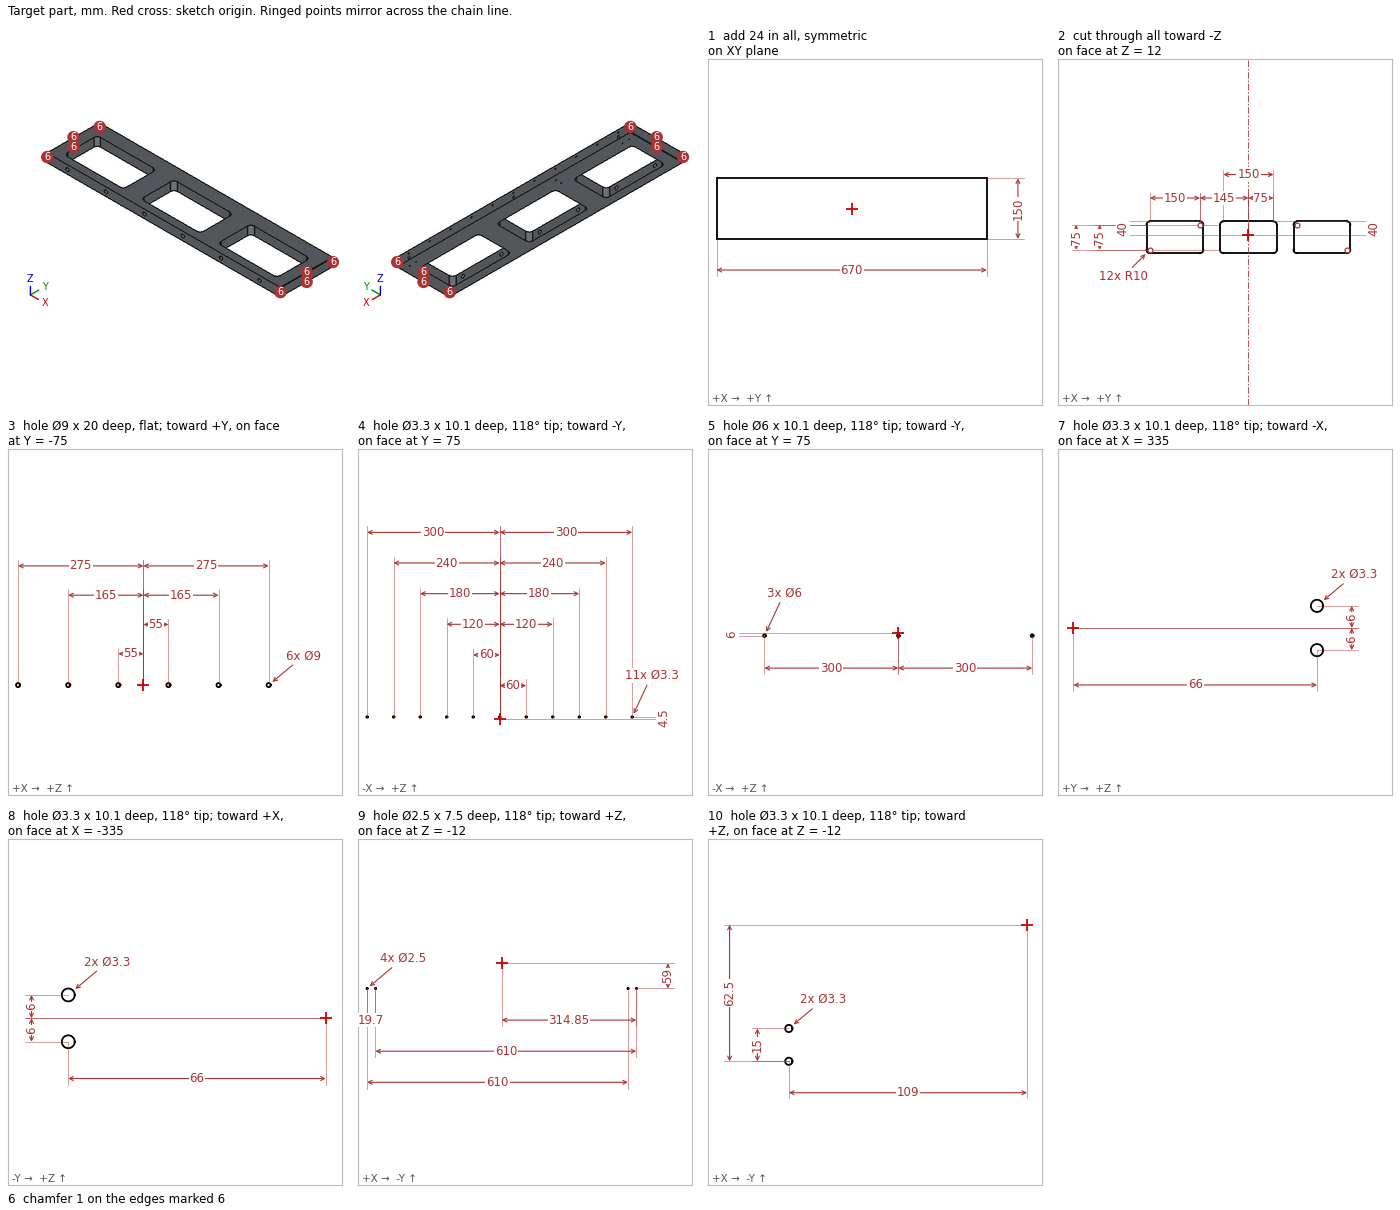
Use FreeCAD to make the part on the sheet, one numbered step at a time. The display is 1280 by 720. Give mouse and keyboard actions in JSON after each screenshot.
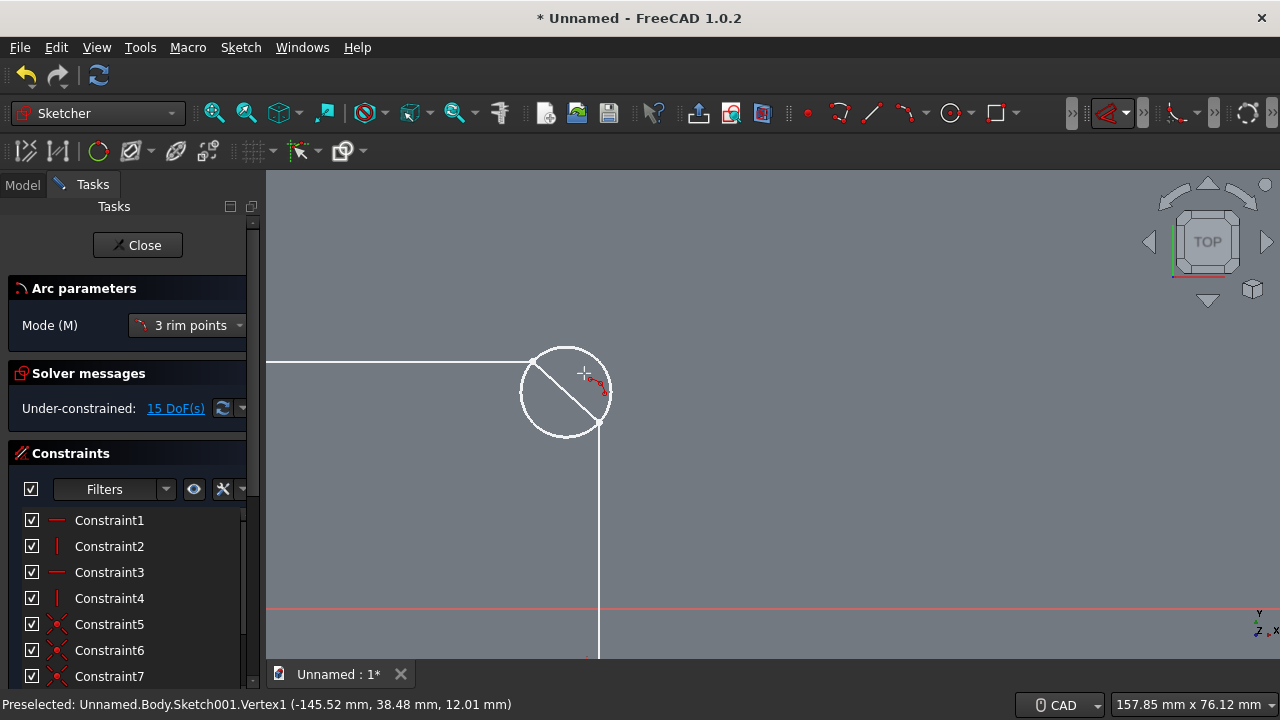
{"action": "left_click", "coordinate": [581, 371]}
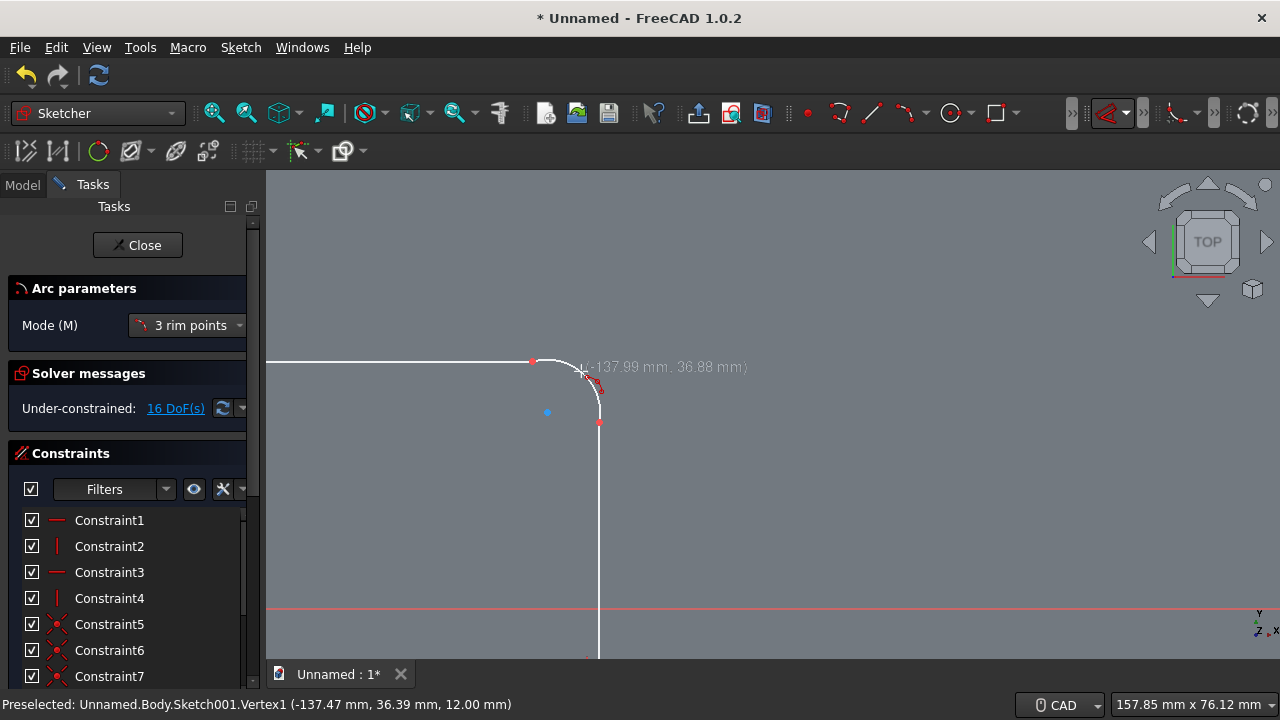
{"action": "left_click", "coordinate": [872, 114]}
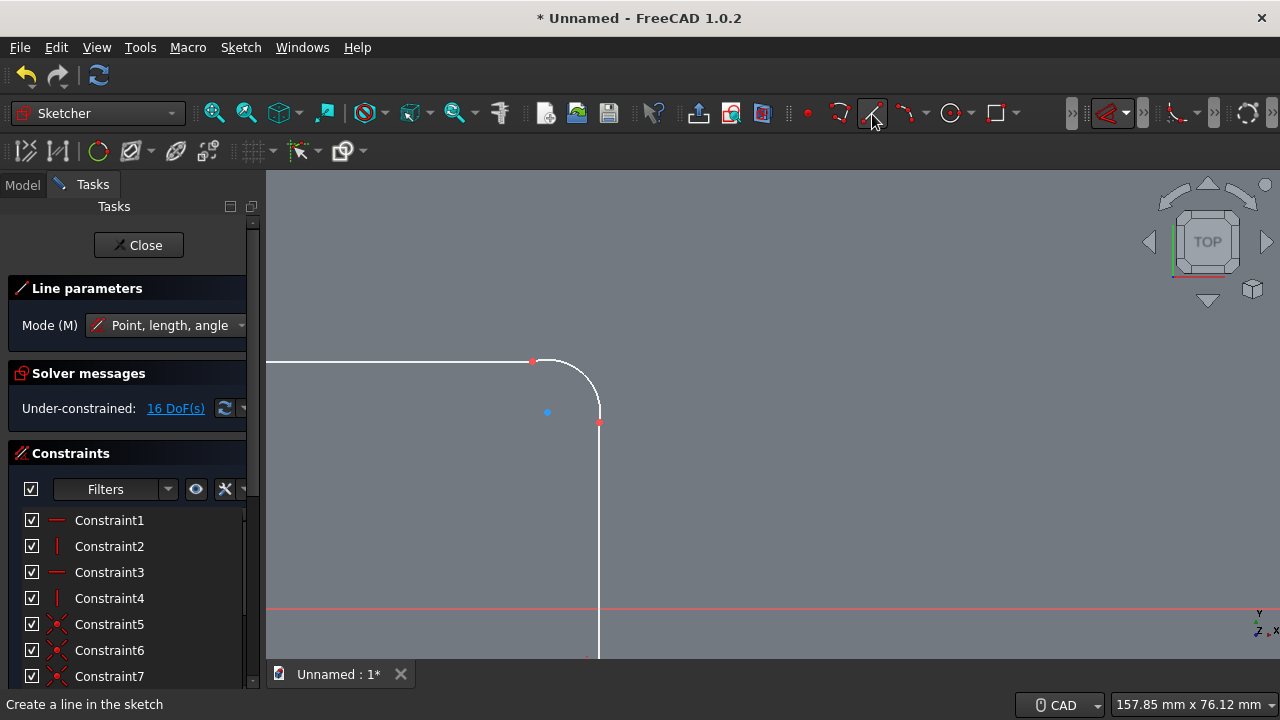
{"action": "scroll", "coordinate": [585, 377], "scroll_direction": "down", "scroll_amount": 10}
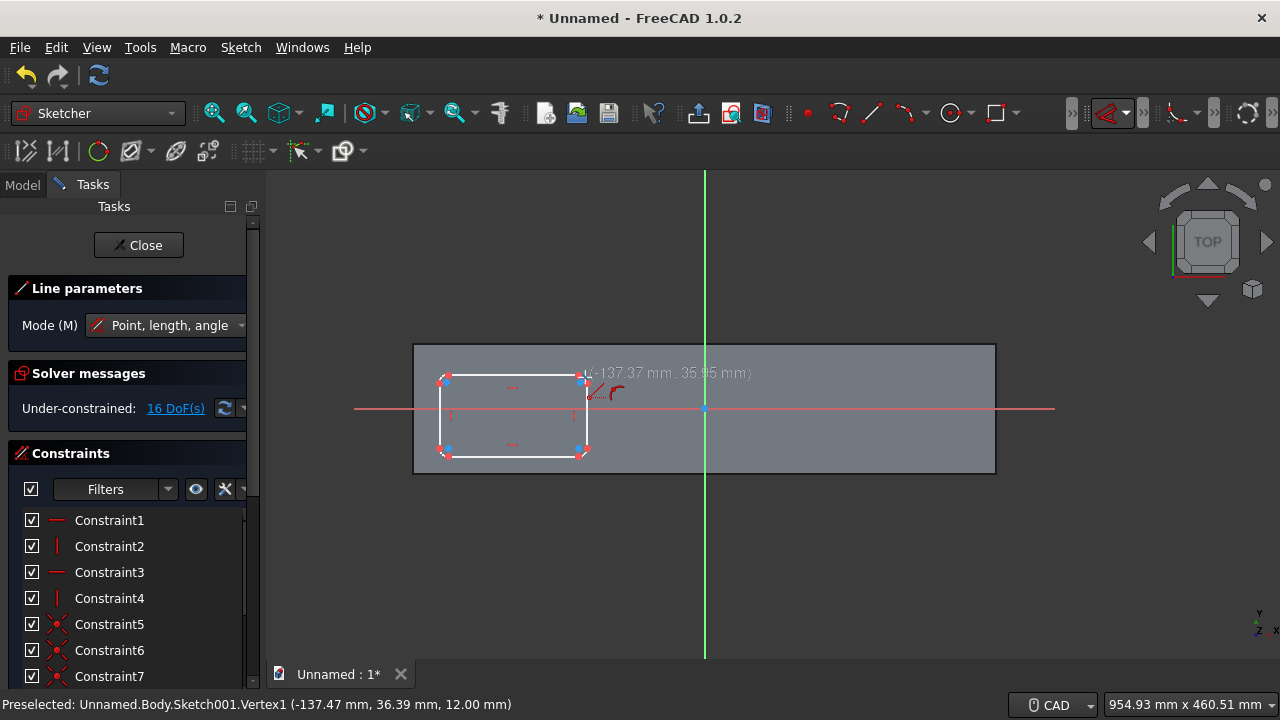
{"action": "left_click", "coordinate": [770, 374]}
{"action": "left_click", "coordinate": [639, 374]}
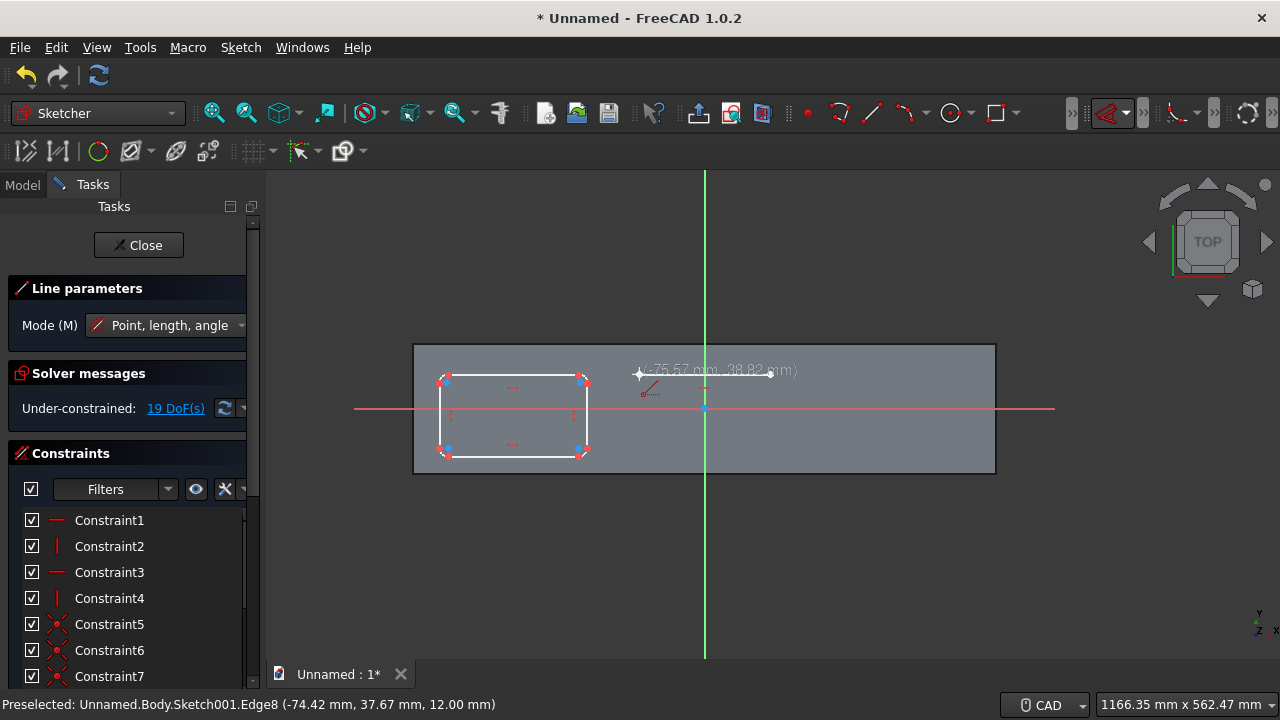
{"action": "scroll", "coordinate": [631, 383], "scroll_direction": "up", "scroll_amount": 2}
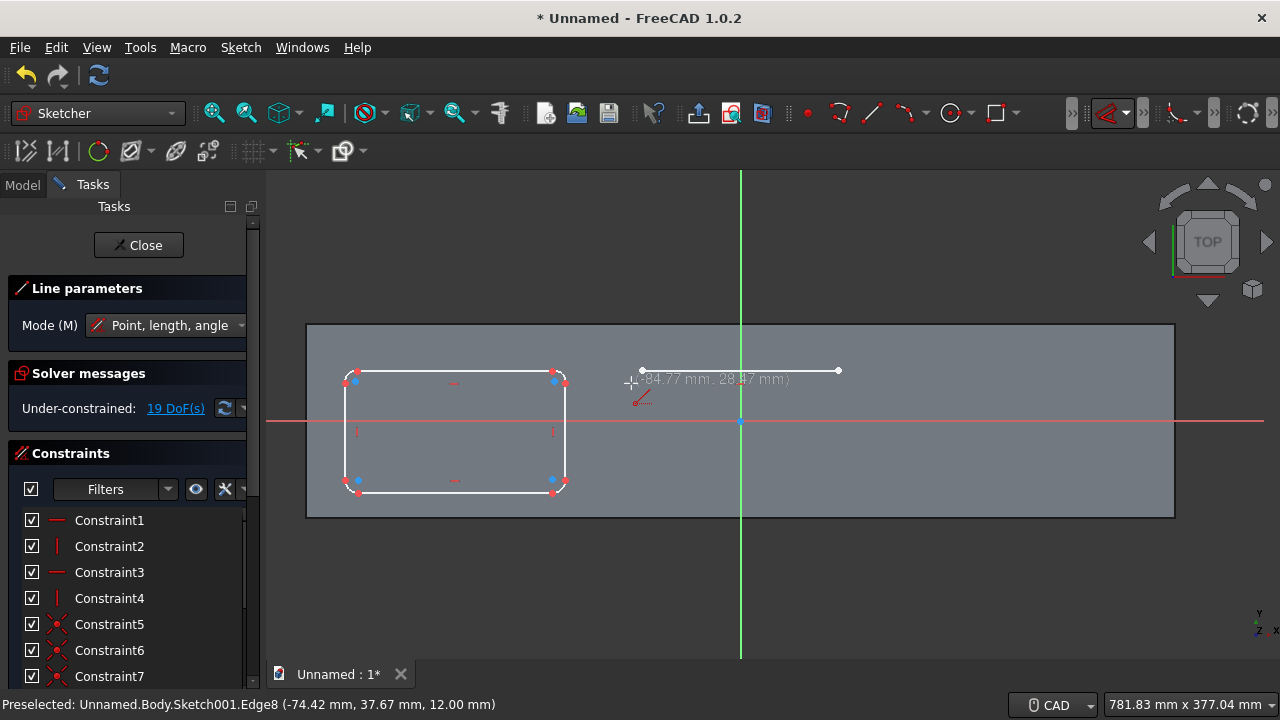
{"action": "left_click", "coordinate": [631, 382]}
{"action": "left_click", "coordinate": [631, 480]}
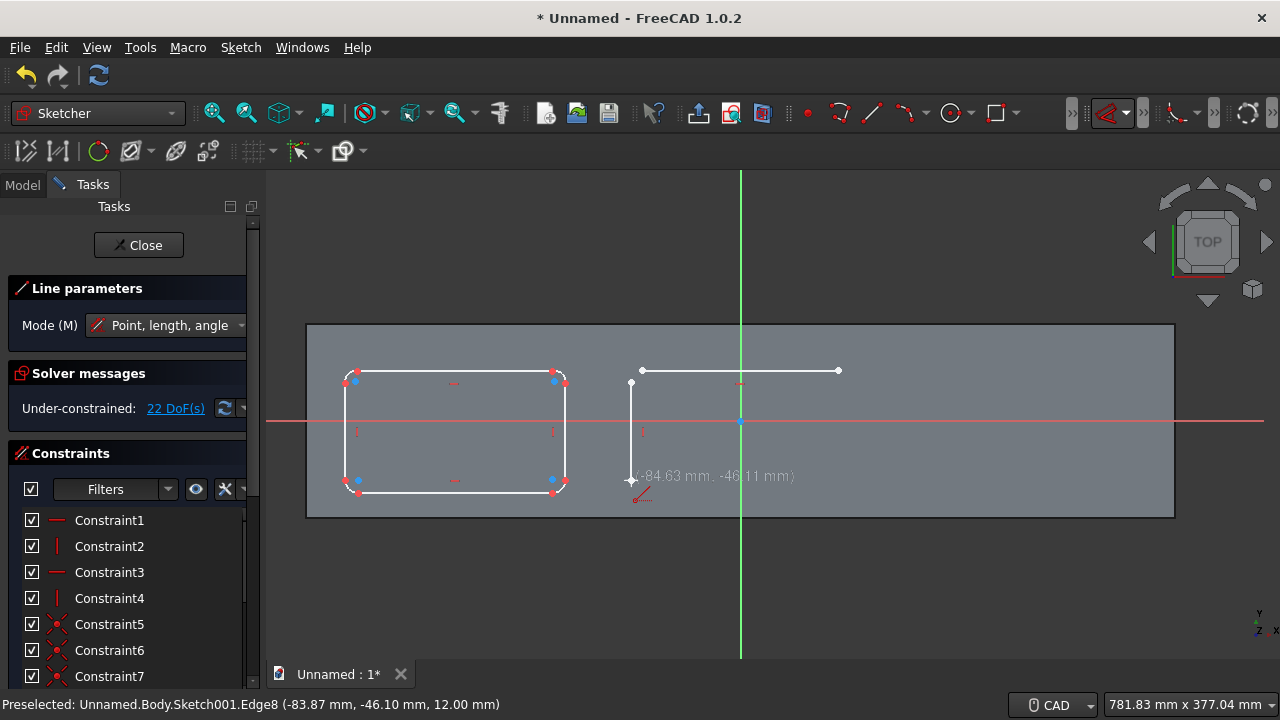
{"action": "left_click", "coordinate": [643, 493]}
{"action": "left_click", "coordinate": [838, 493]}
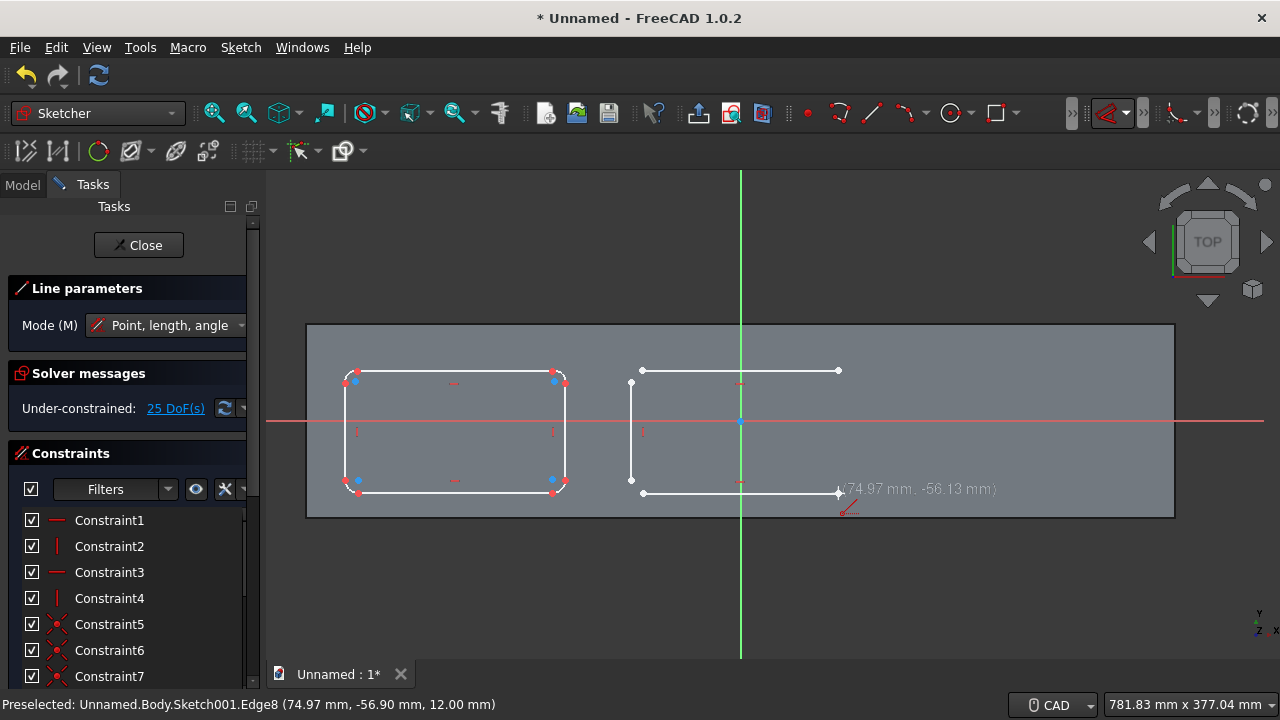
{"action": "left_click", "coordinate": [851, 480]}
{"action": "left_click", "coordinate": [851, 382]}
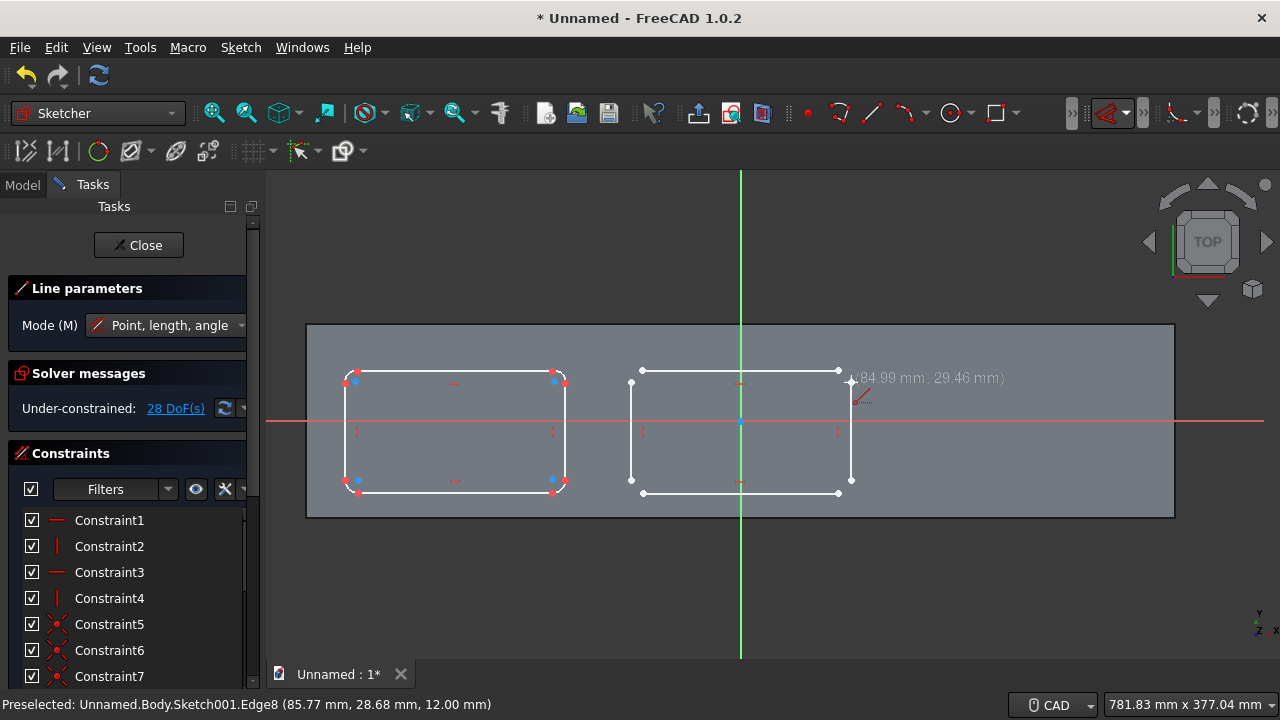
{"action": "left_click", "coordinate": [906, 114]}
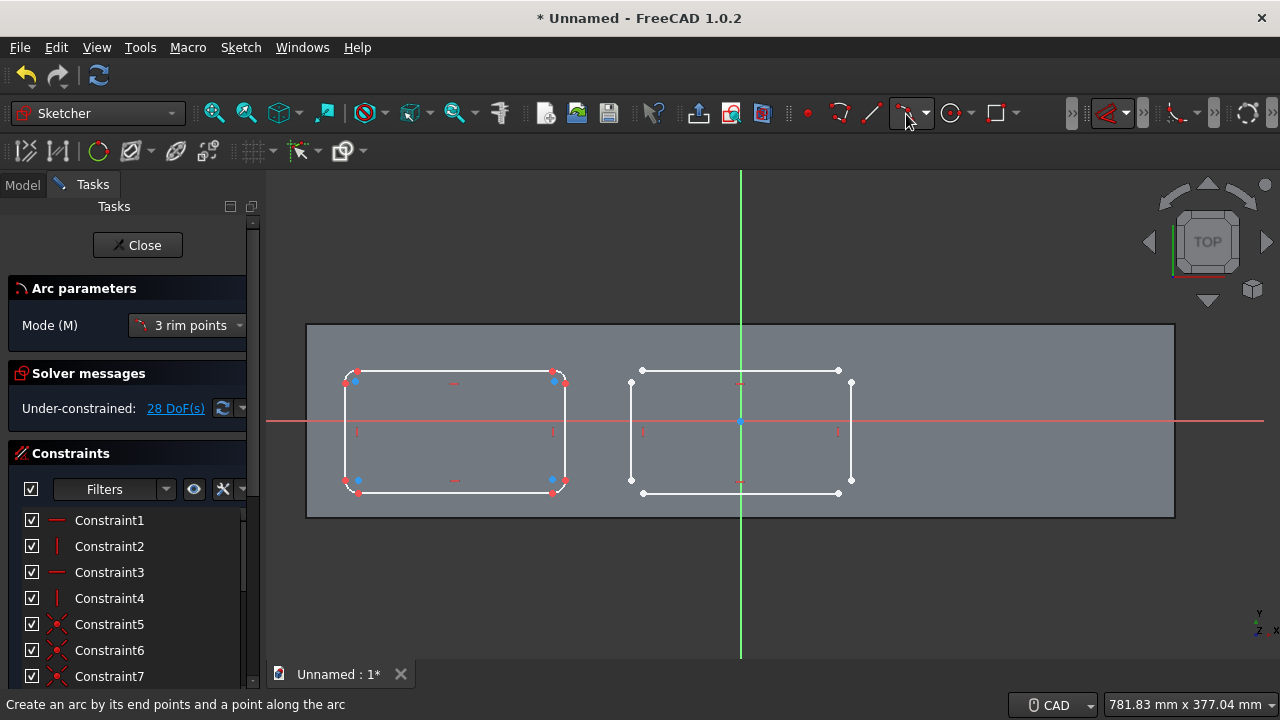
{"action": "left_click", "coordinate": [643, 371]}
{"action": "left_click", "coordinate": [631, 383]}